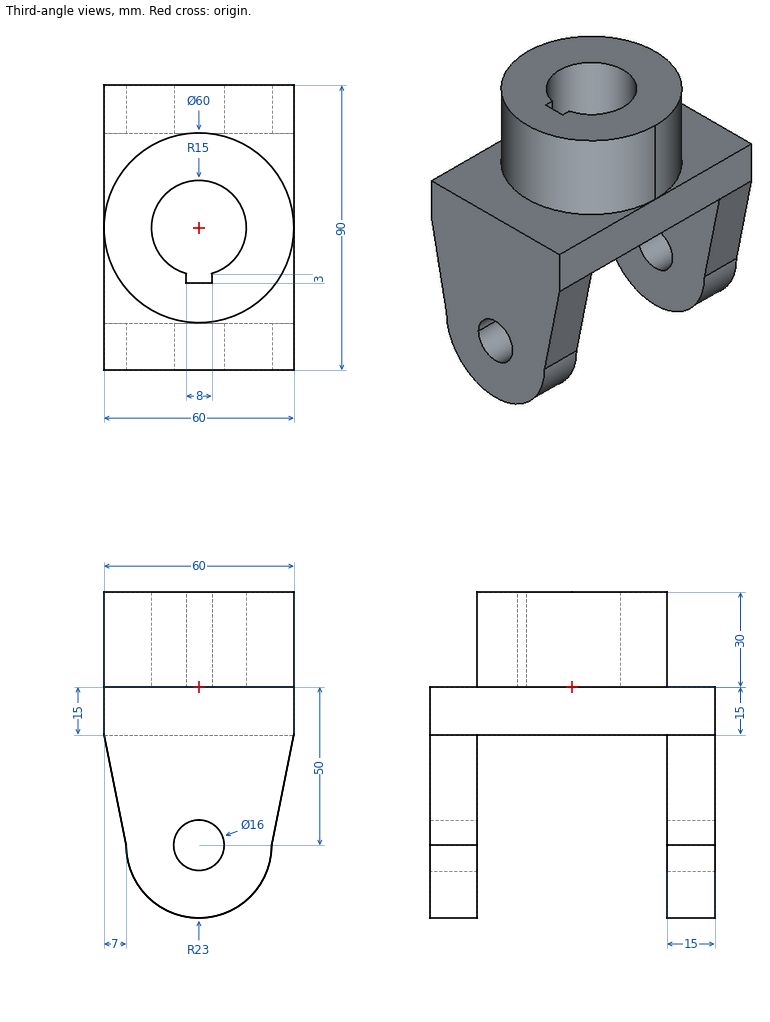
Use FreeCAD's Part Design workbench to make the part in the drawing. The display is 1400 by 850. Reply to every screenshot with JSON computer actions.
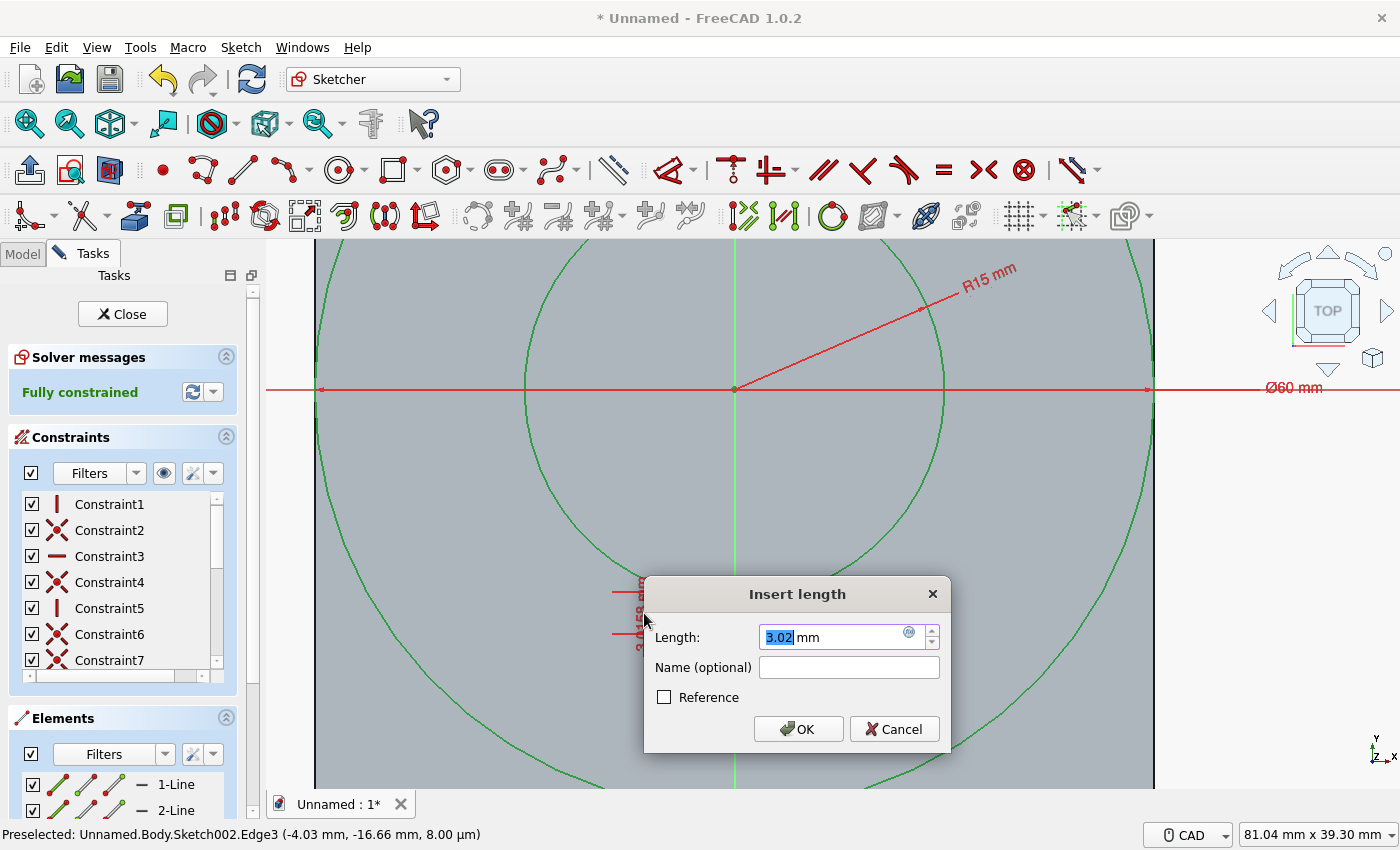
{"action": "type", "text": "3"}
{"action": "key", "text": "Return"}
{"action": "key", "text": "Escape"}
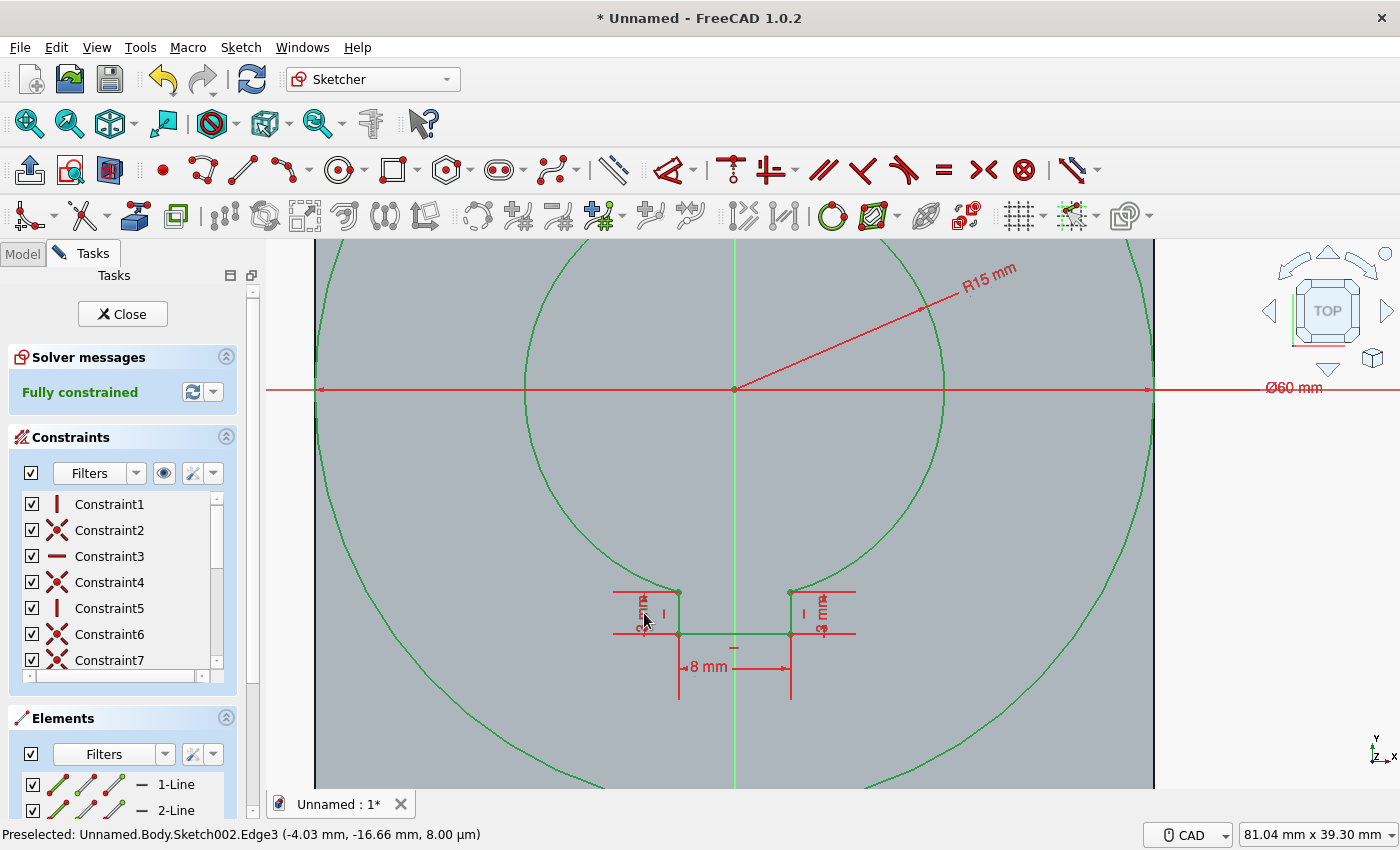
{"action": "left_click", "coordinate": [123, 314]}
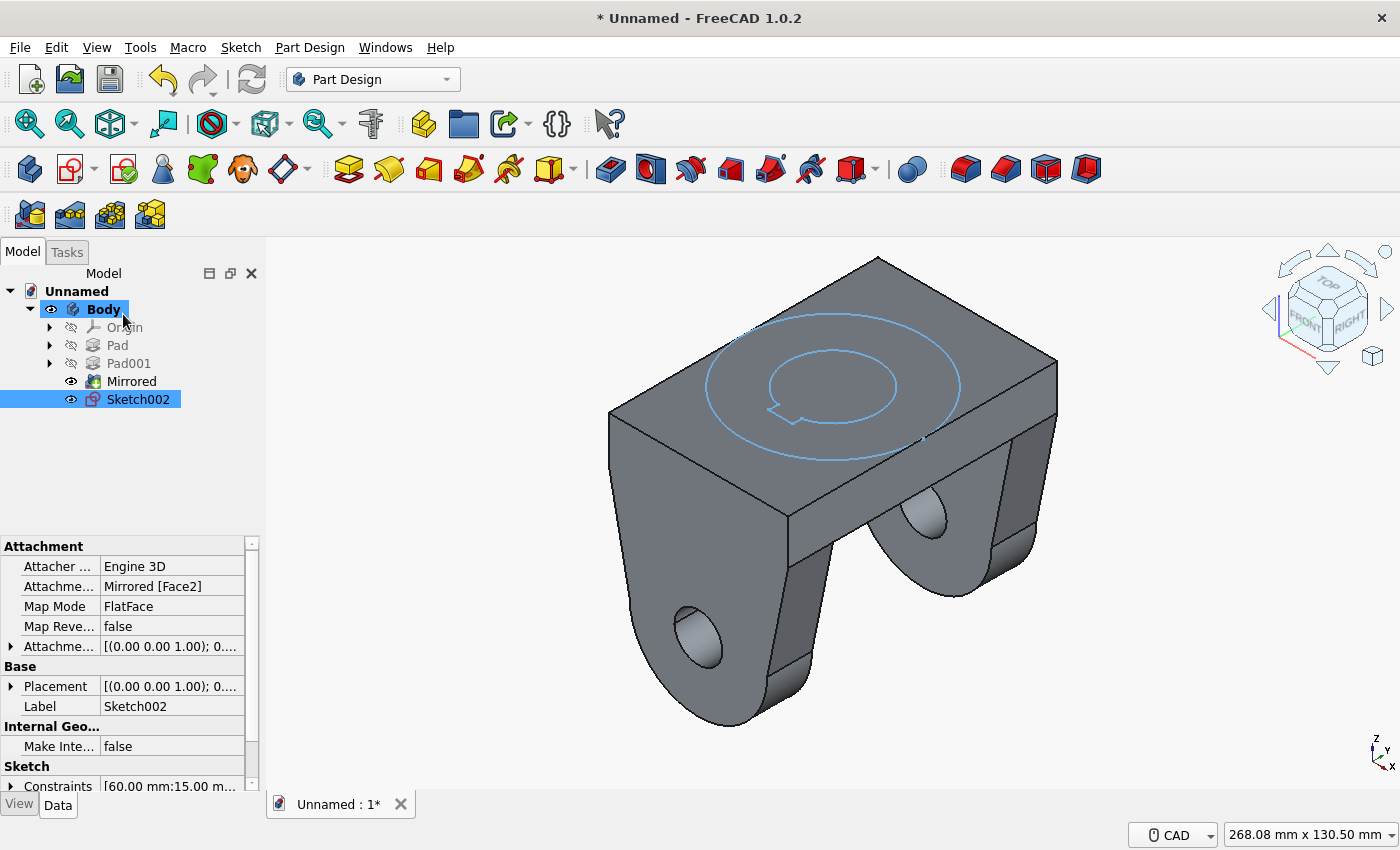
{"action": "left_click", "coordinate": [350, 170]}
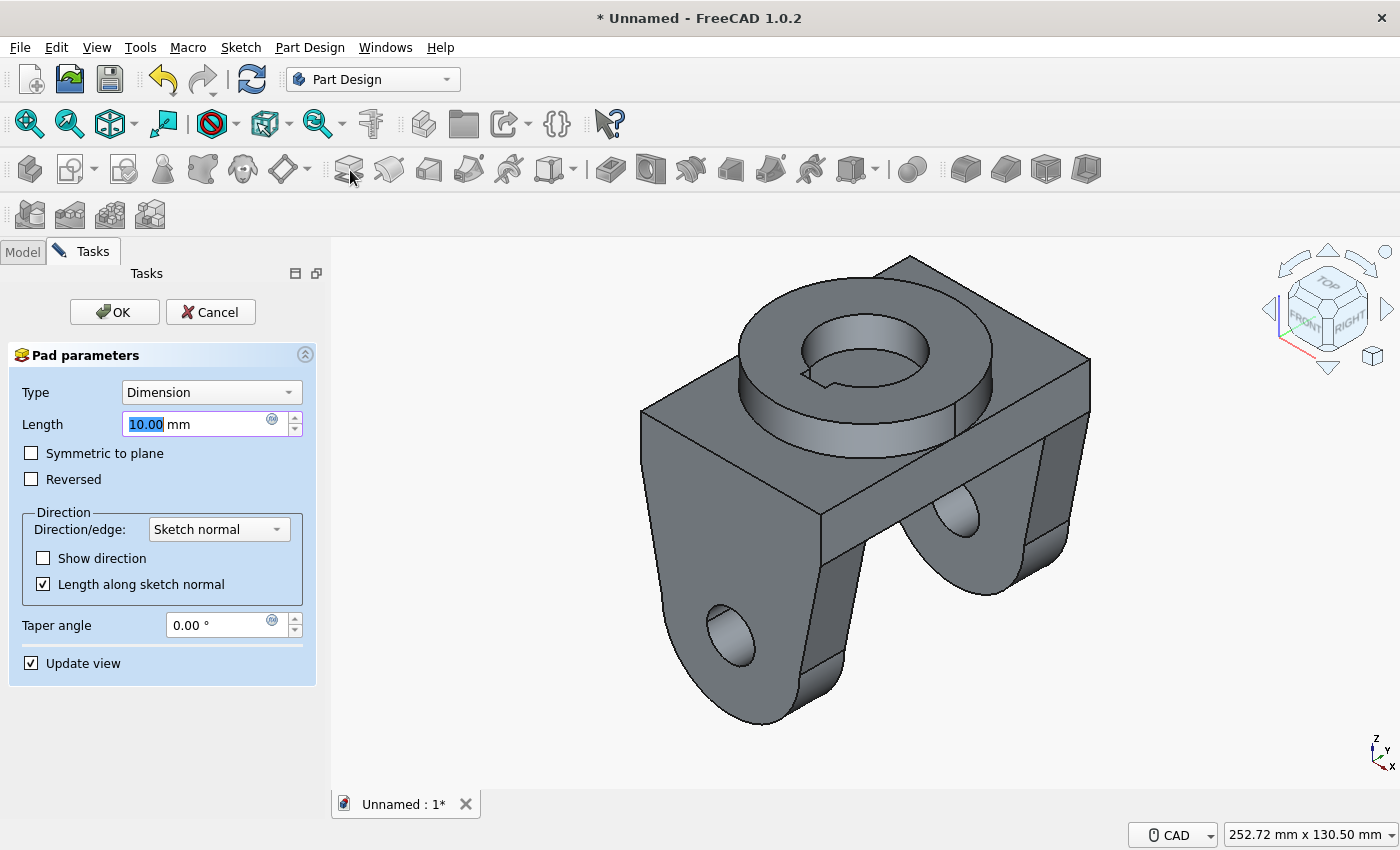
{"action": "type", "text": "30"}
{"action": "key", "text": "Tab"}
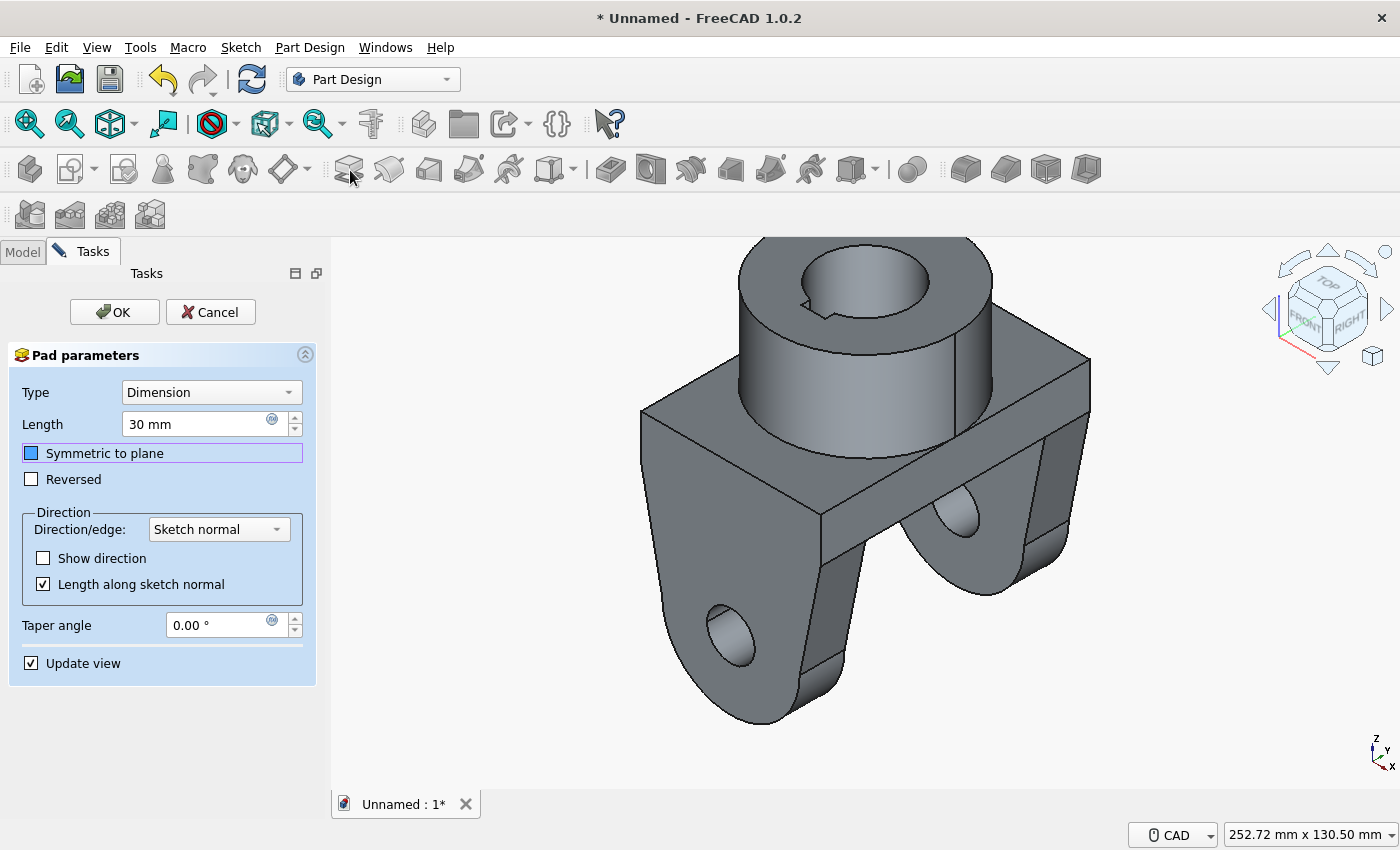
{"action": "left_click", "coordinate": [115, 312]}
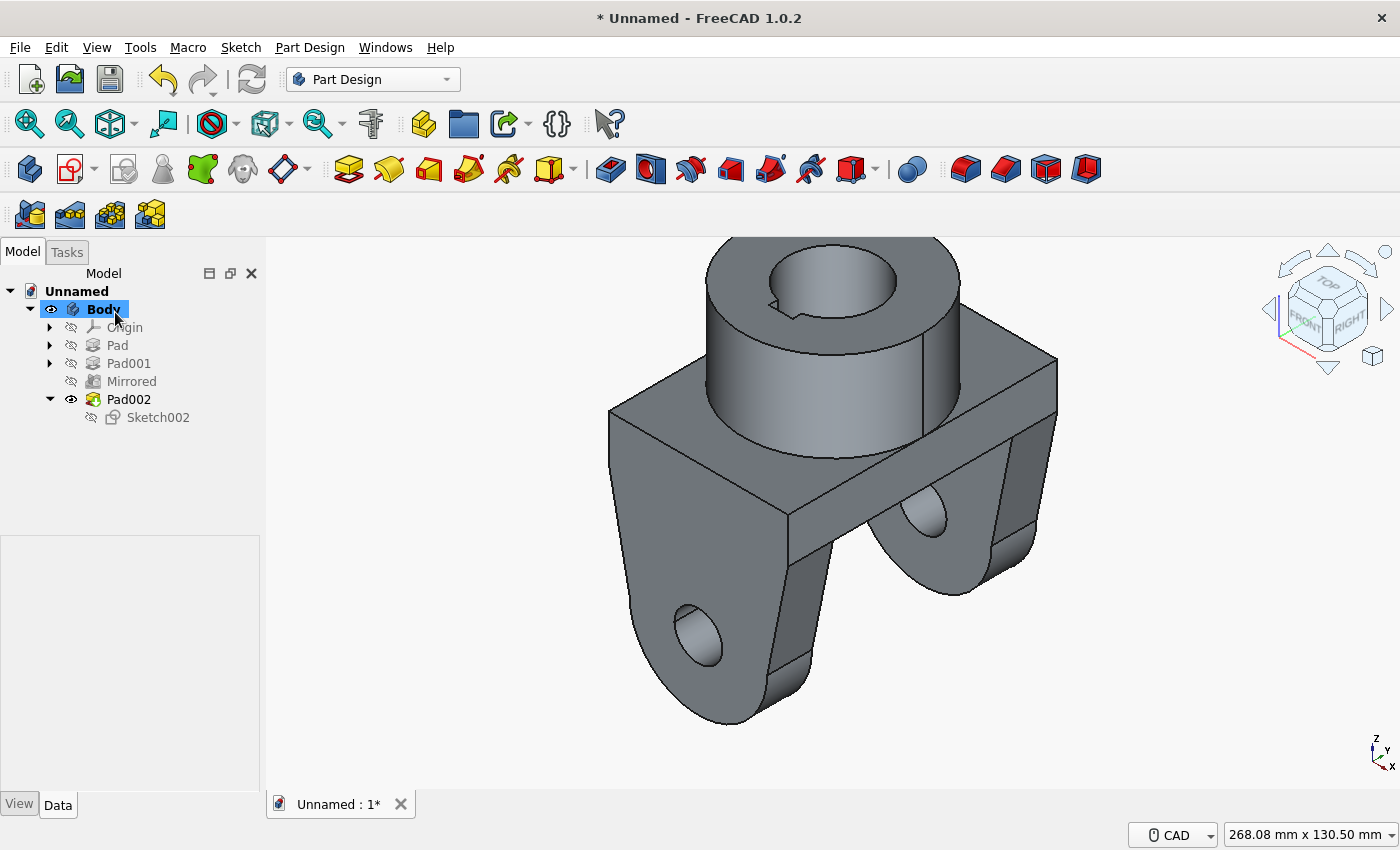
{"action": "left_click", "coordinate": [30, 124]}